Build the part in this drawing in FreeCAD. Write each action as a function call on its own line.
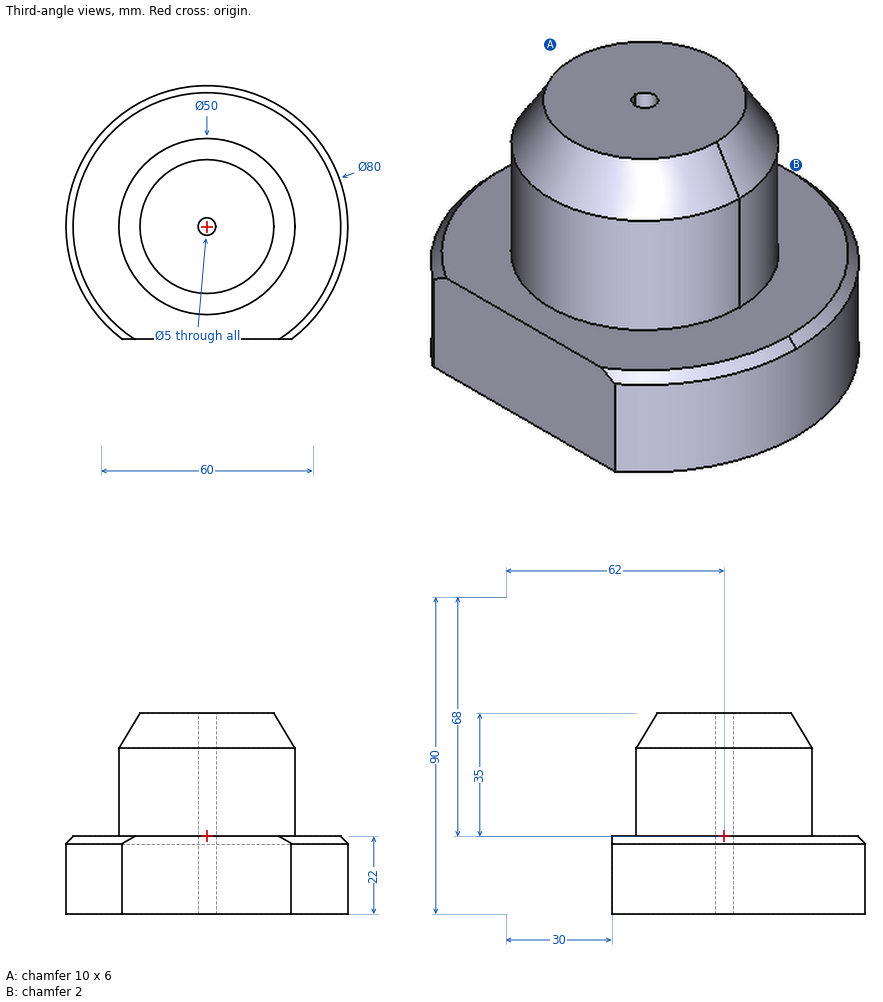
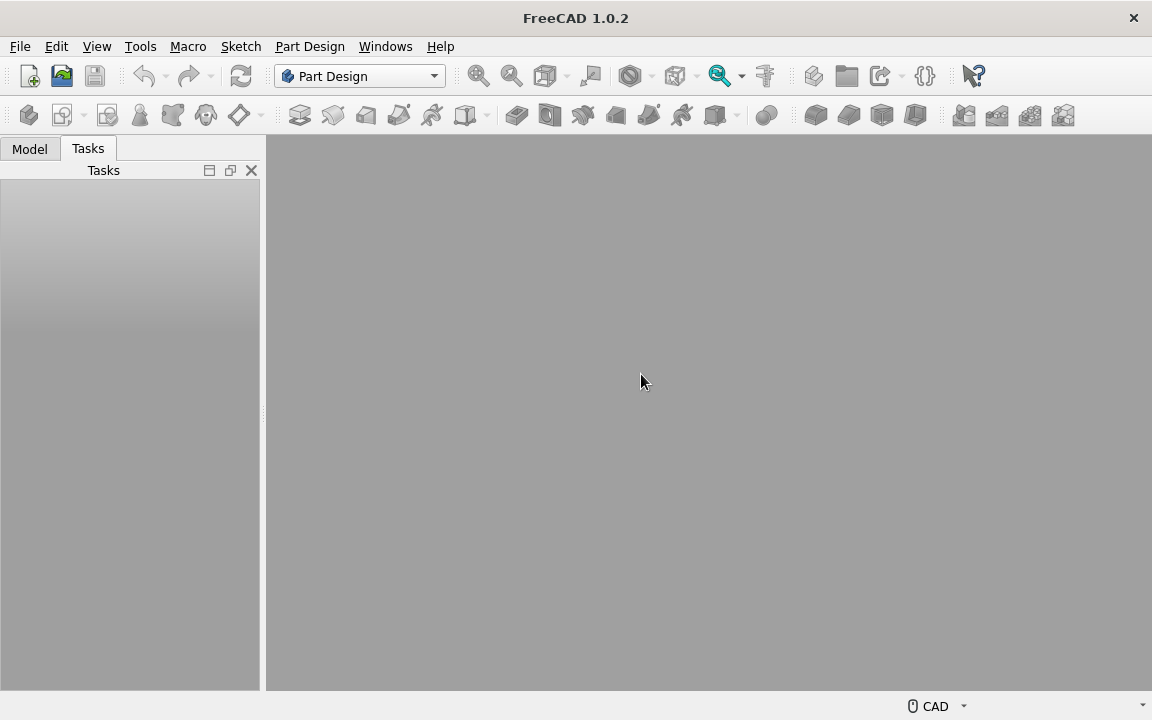
click(29, 76)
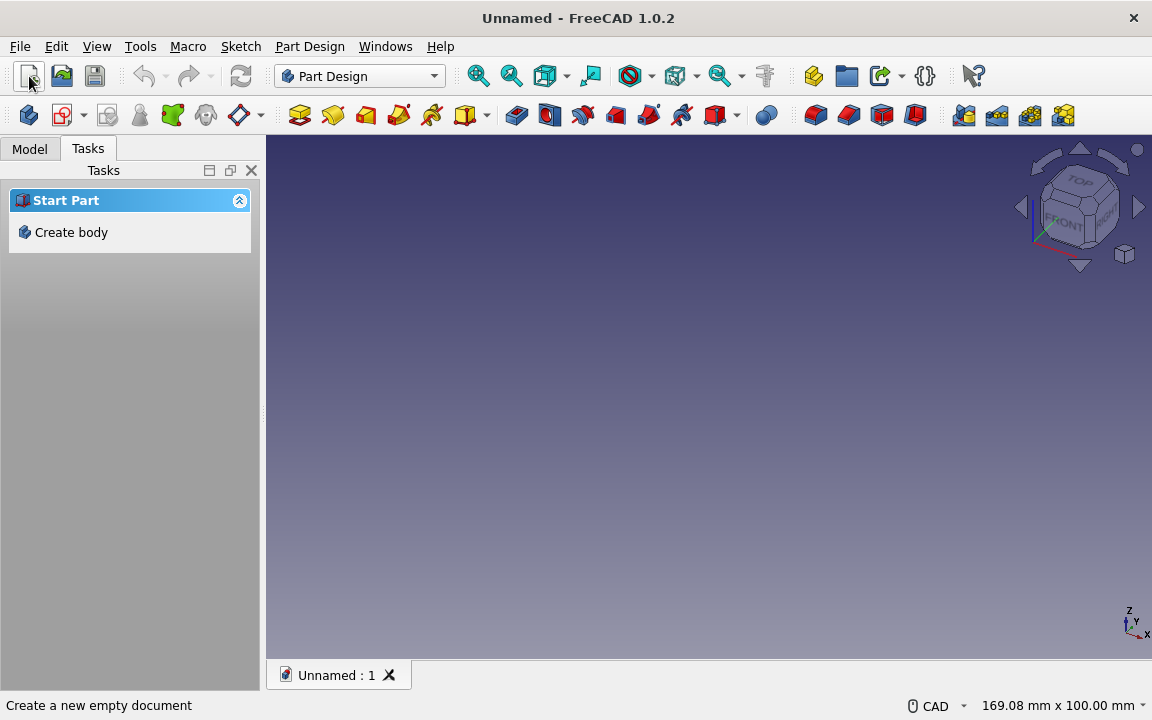
click(62, 116)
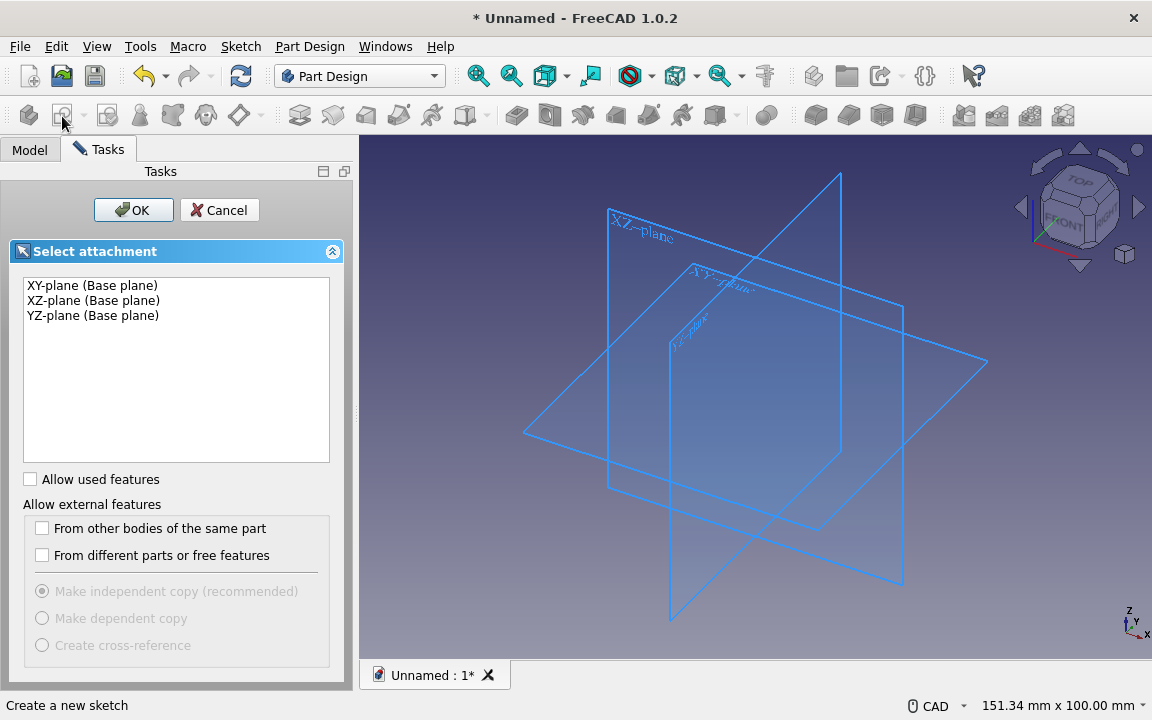
click(84, 286)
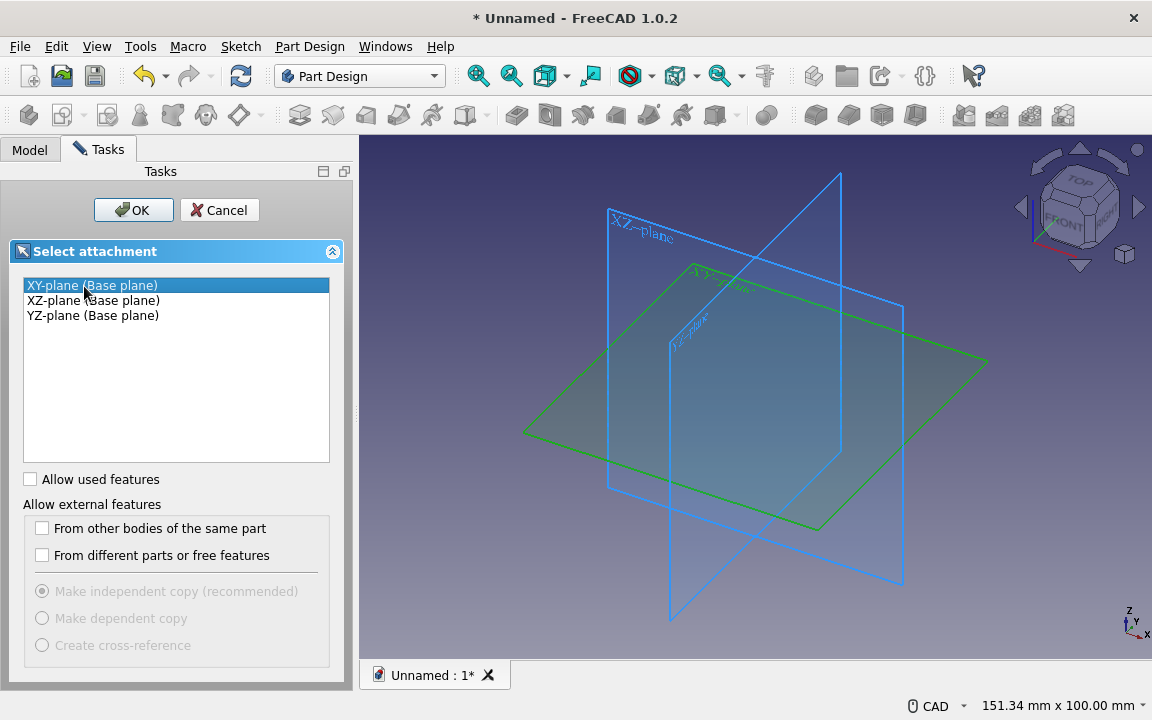
click(134, 210)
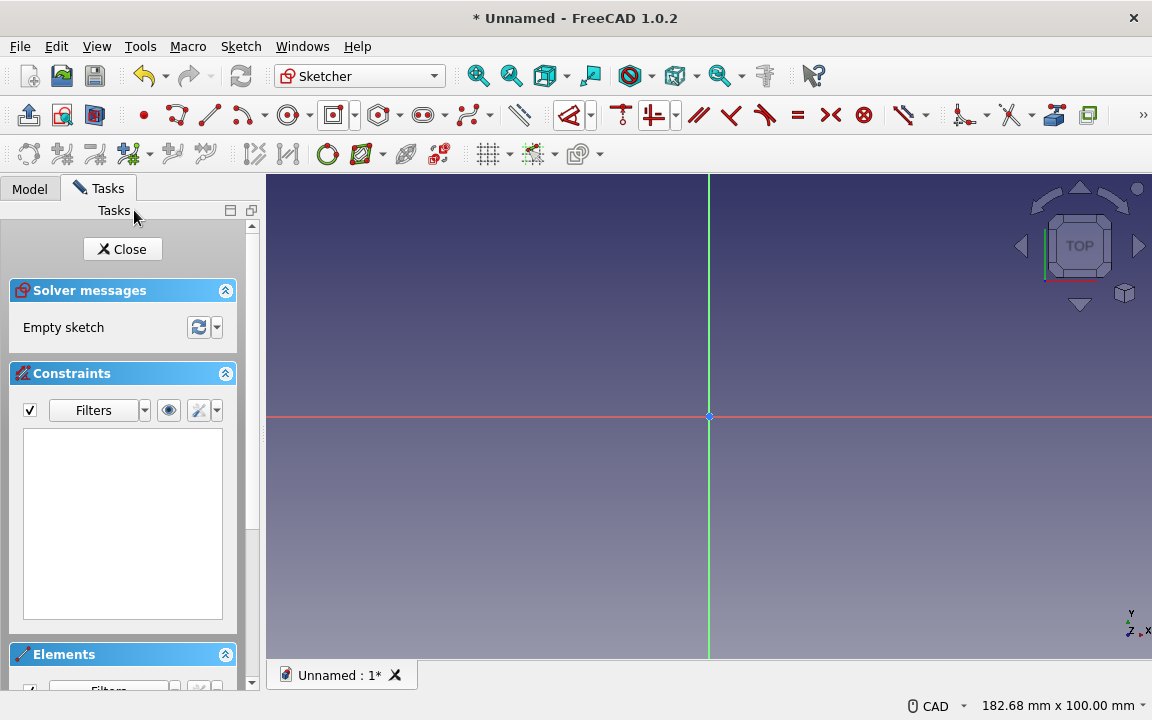
click(288, 116)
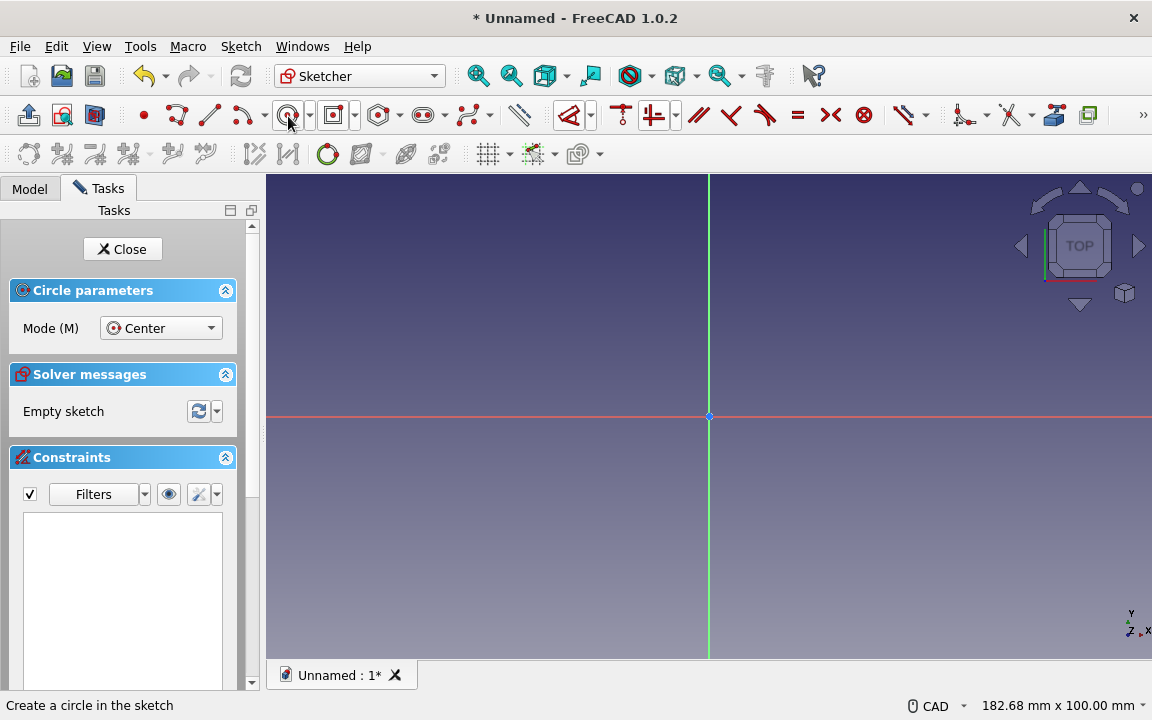
click(709, 416)
click(795, 331)
key(Escape)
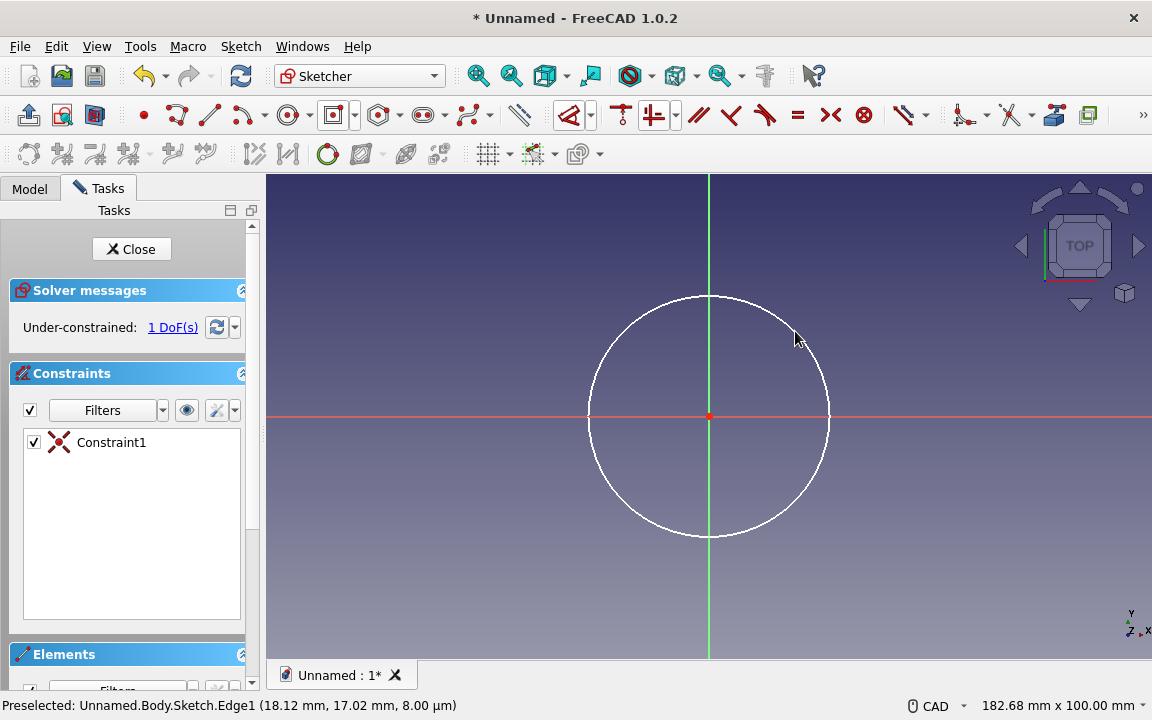
click(568, 116)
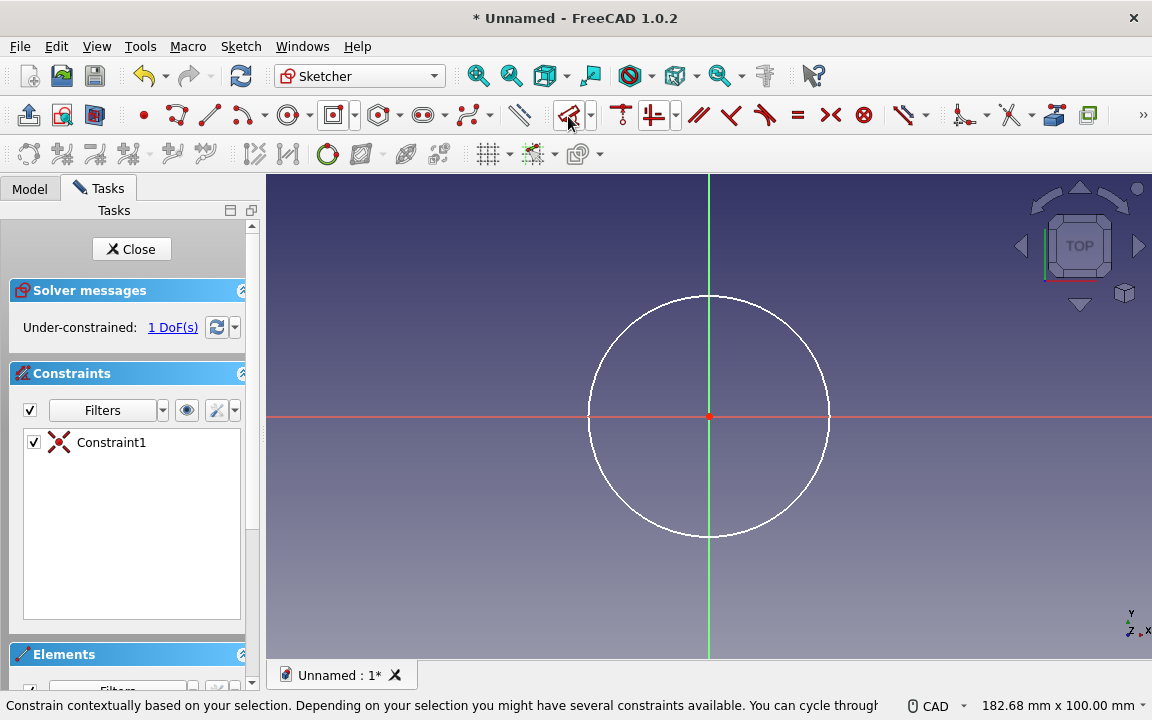
click(794, 331)
click(817, 308)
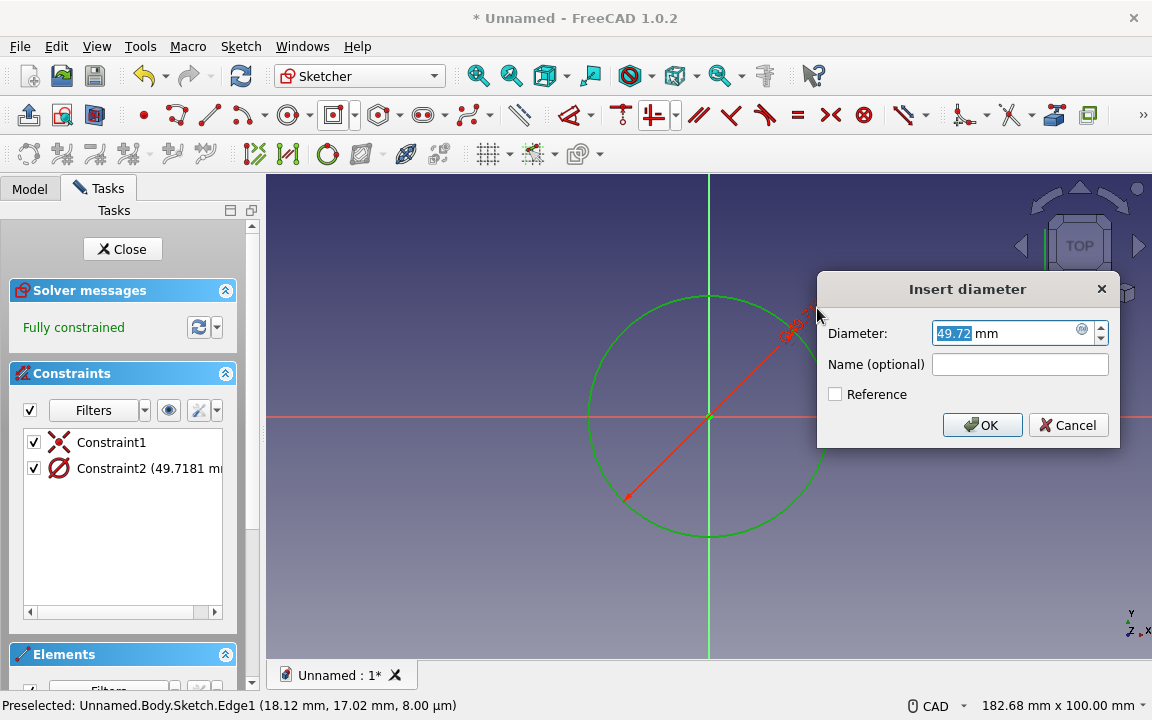
text(50)
key(Return)
key(Escape)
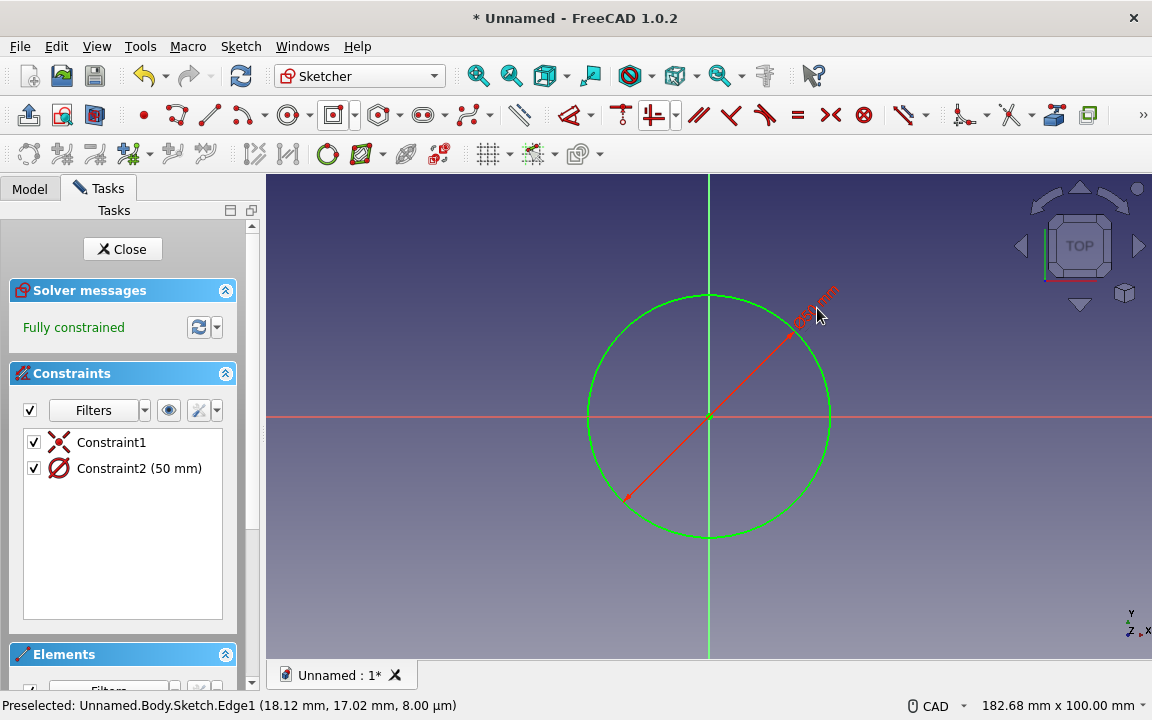
click(123, 249)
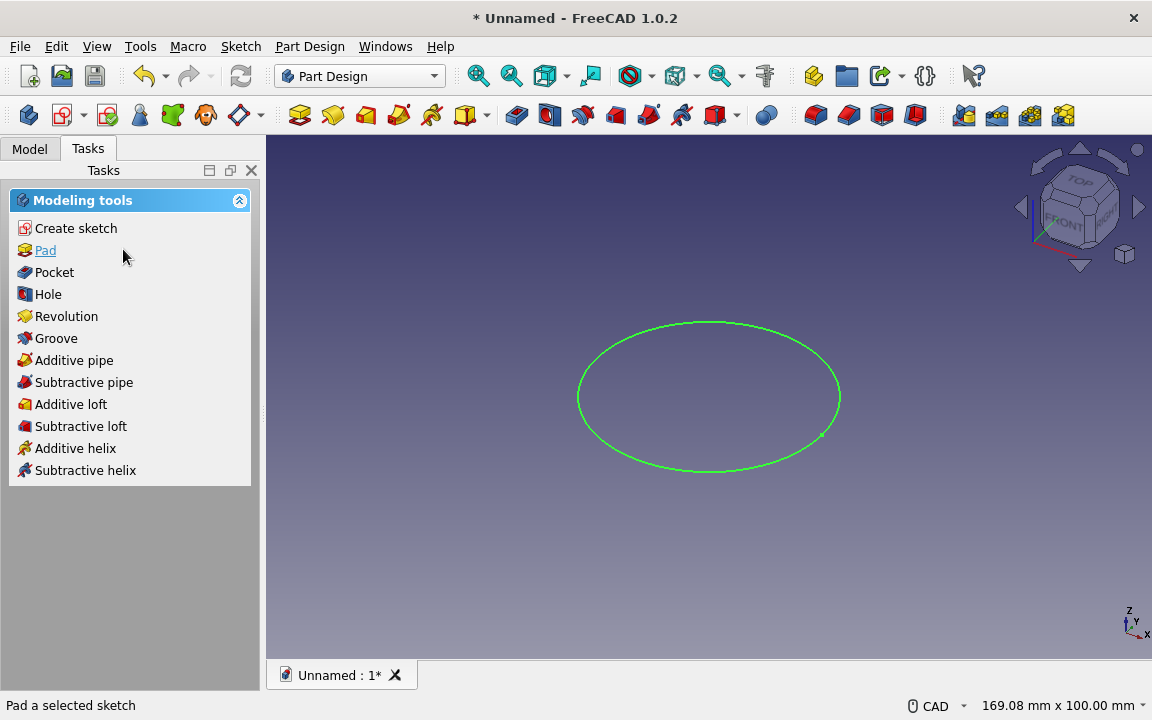
click(300, 116)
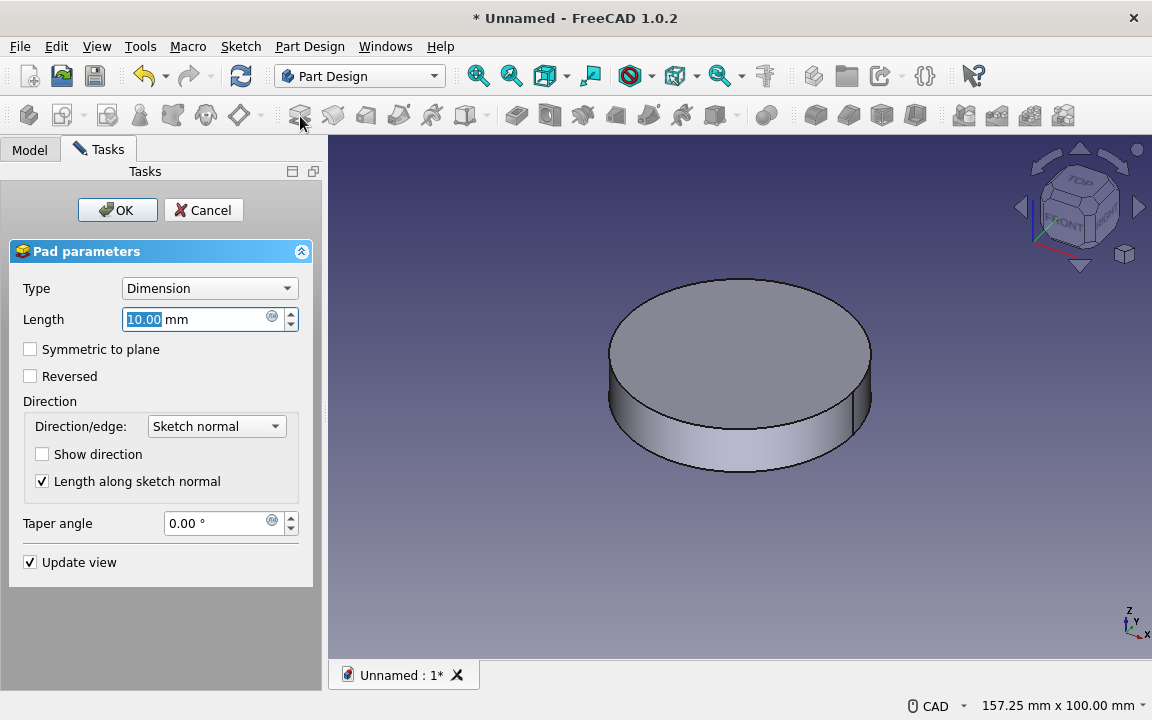
text(35)
key(Tab)